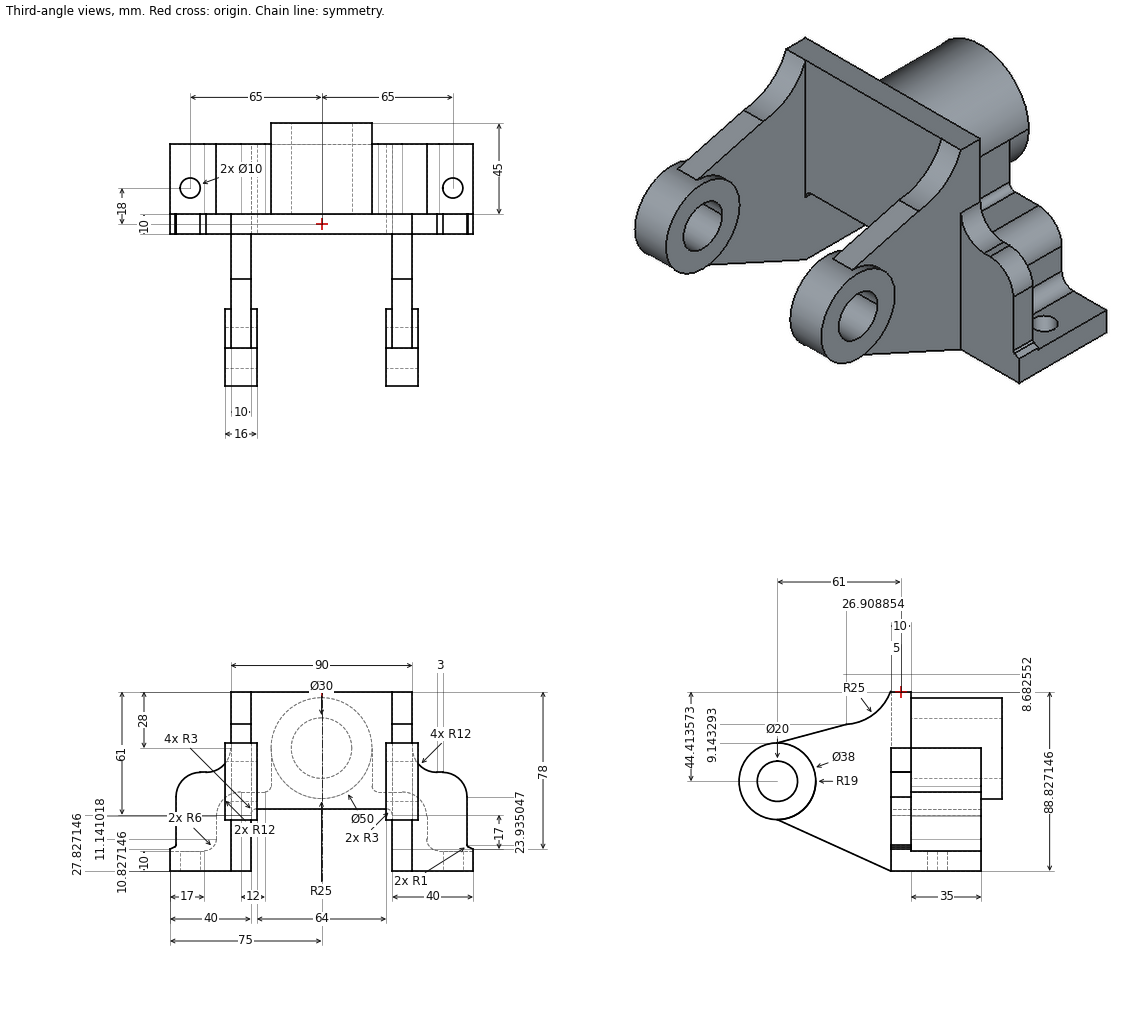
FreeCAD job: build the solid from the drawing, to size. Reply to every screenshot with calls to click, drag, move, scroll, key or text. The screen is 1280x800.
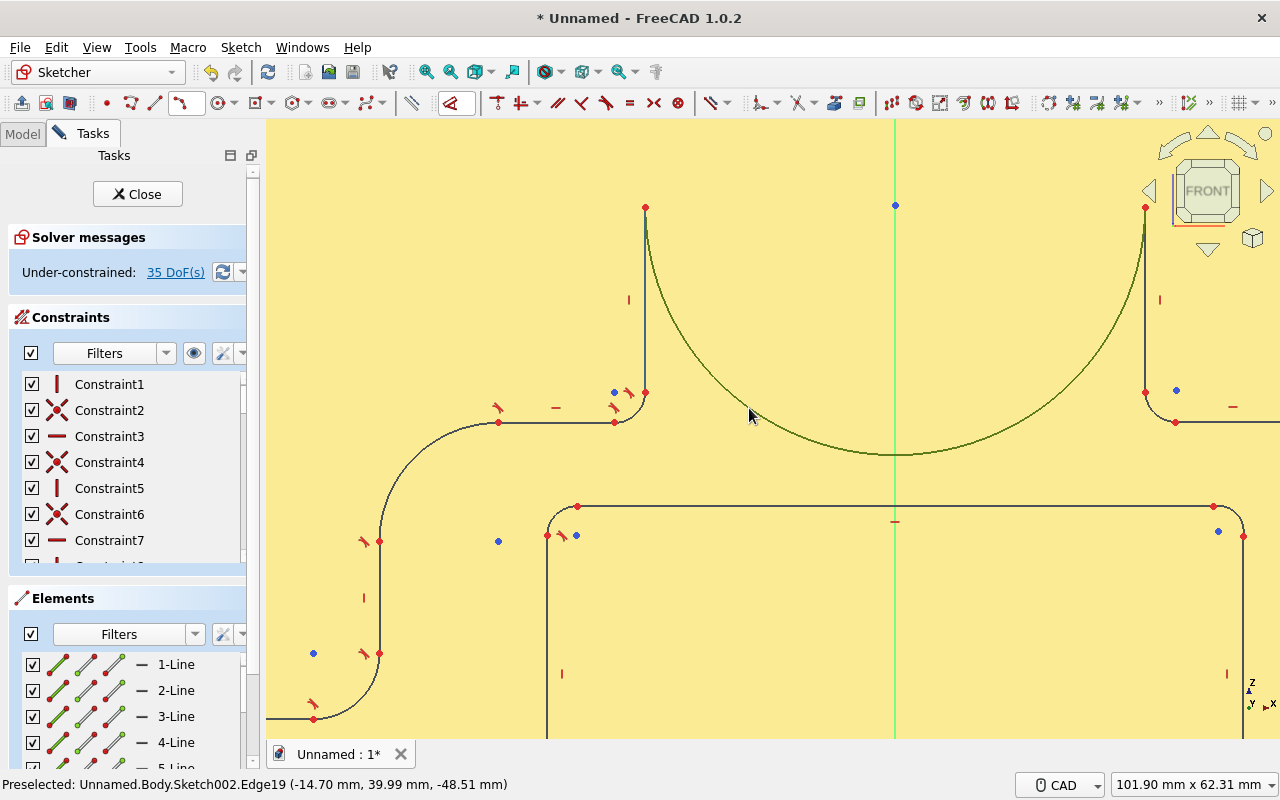
key(t)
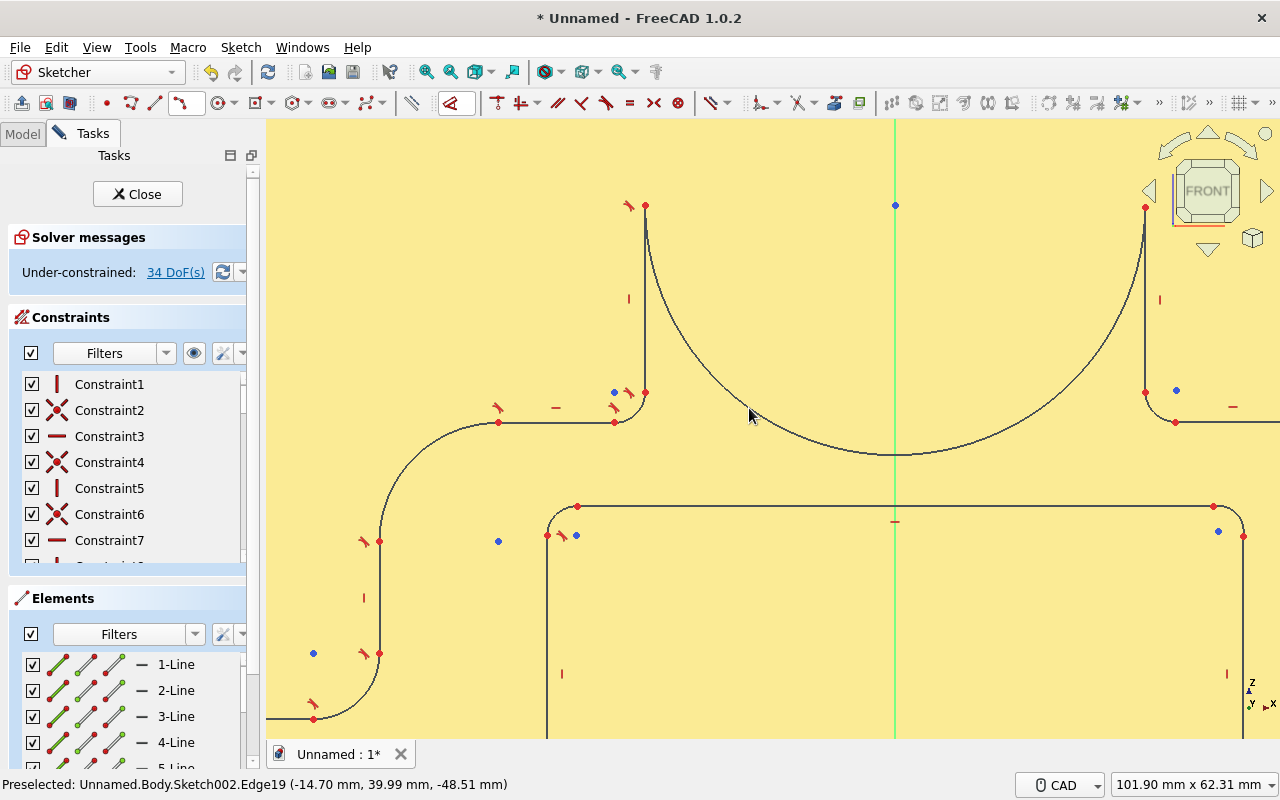
scroll(594, 465, down, 5)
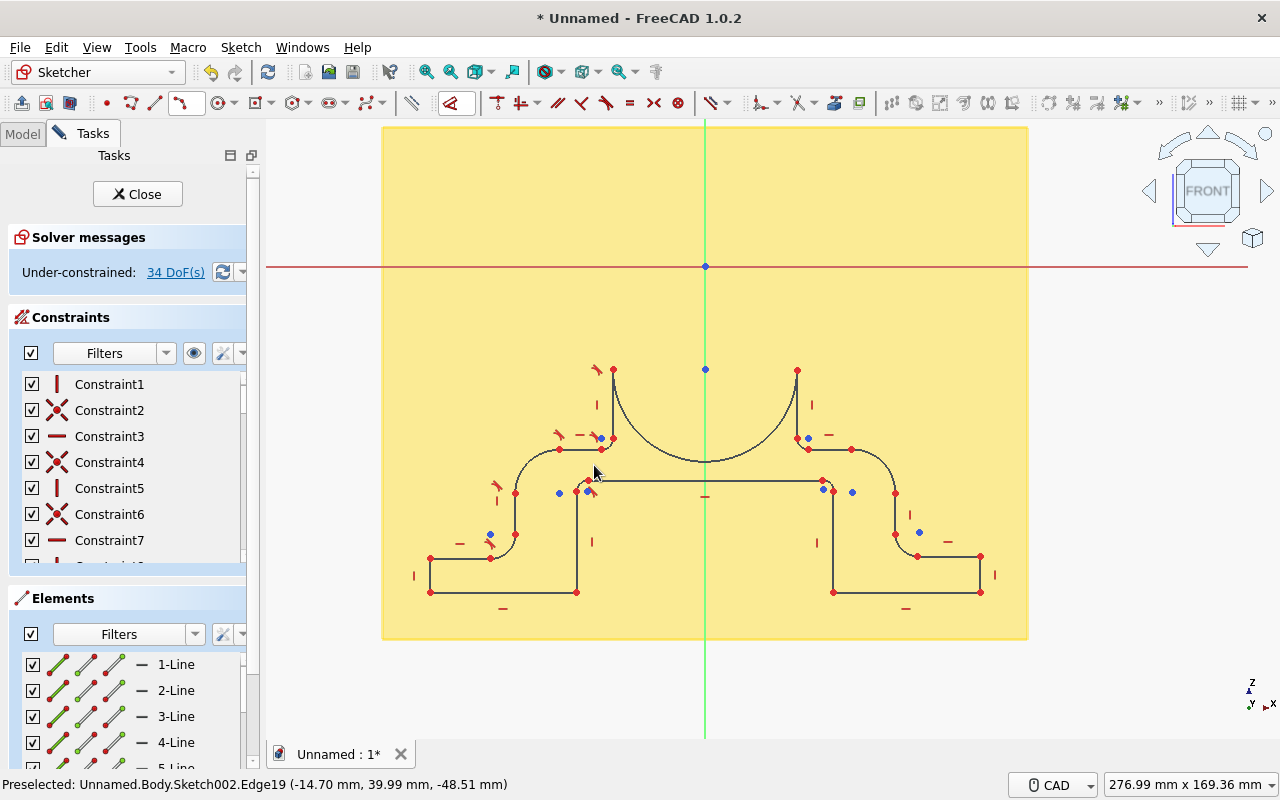
click(797, 418)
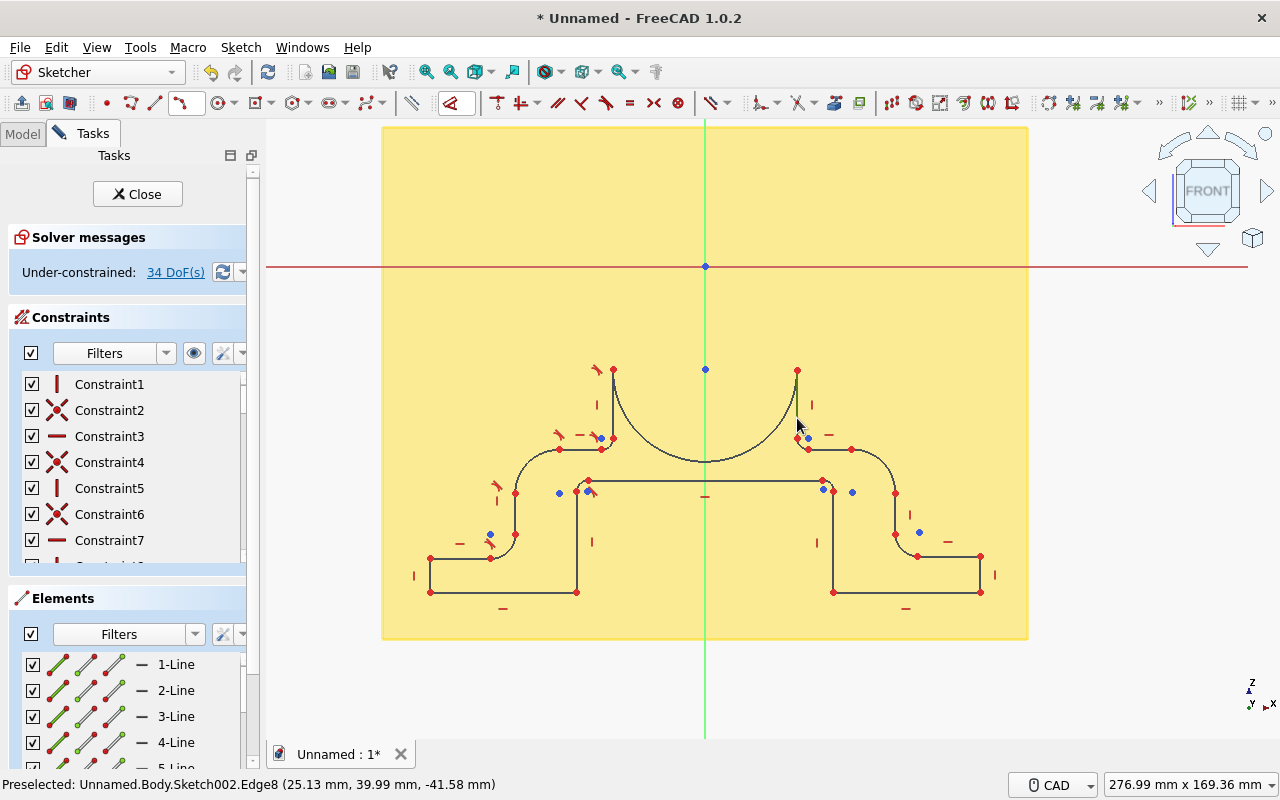
click(651, 444)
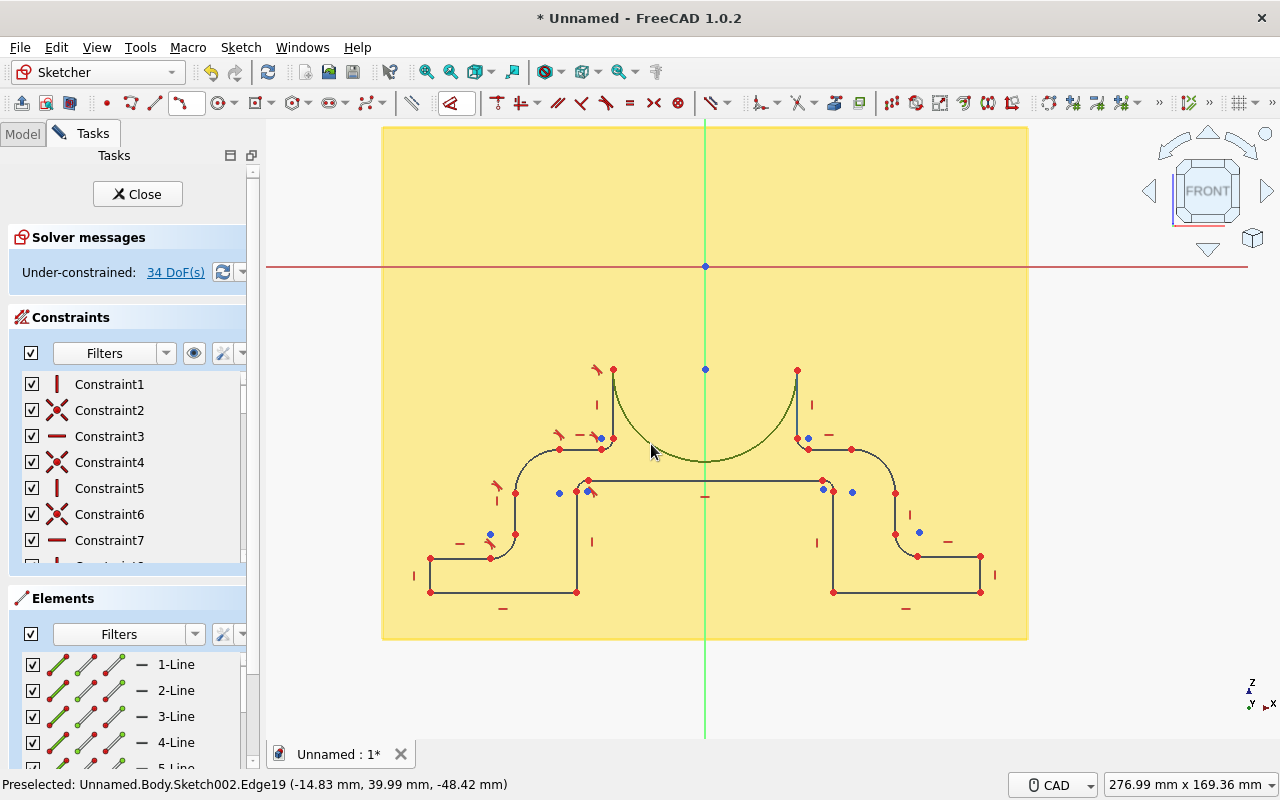
click(606, 104)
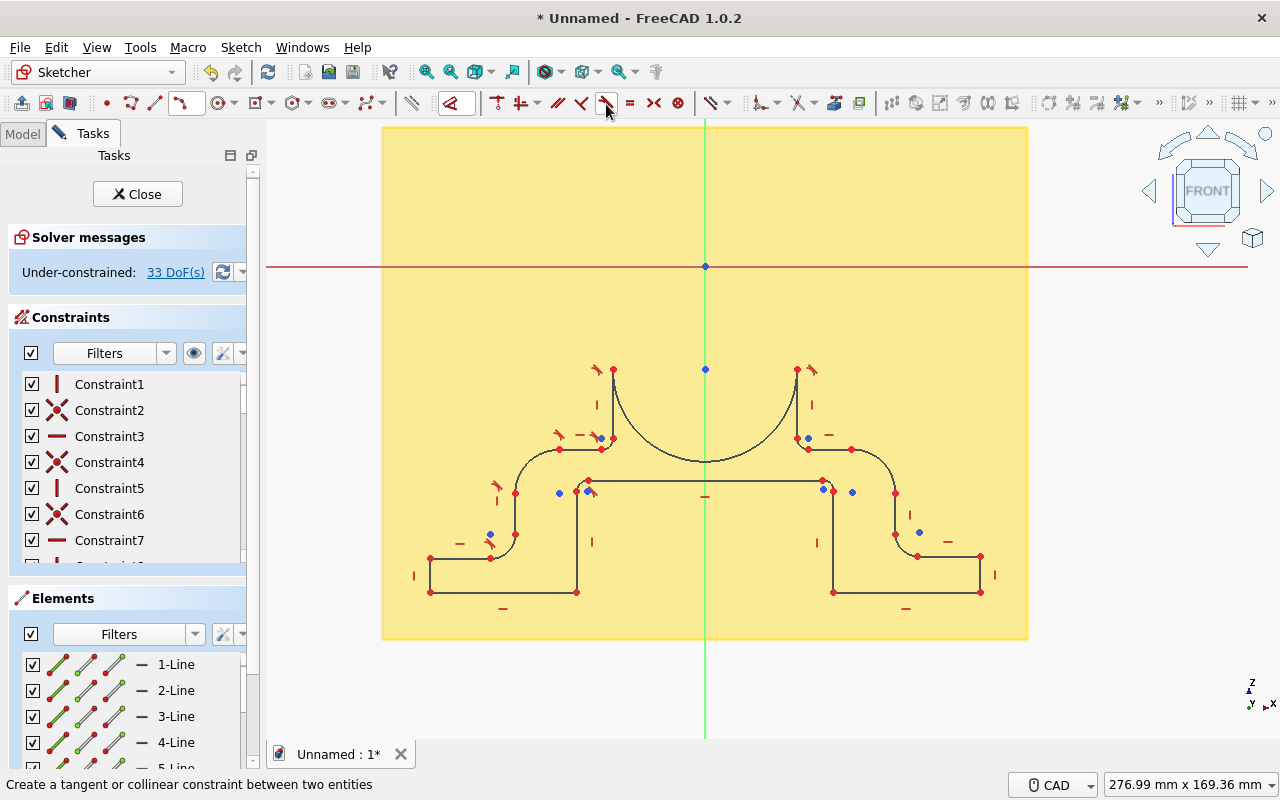
click(797, 418)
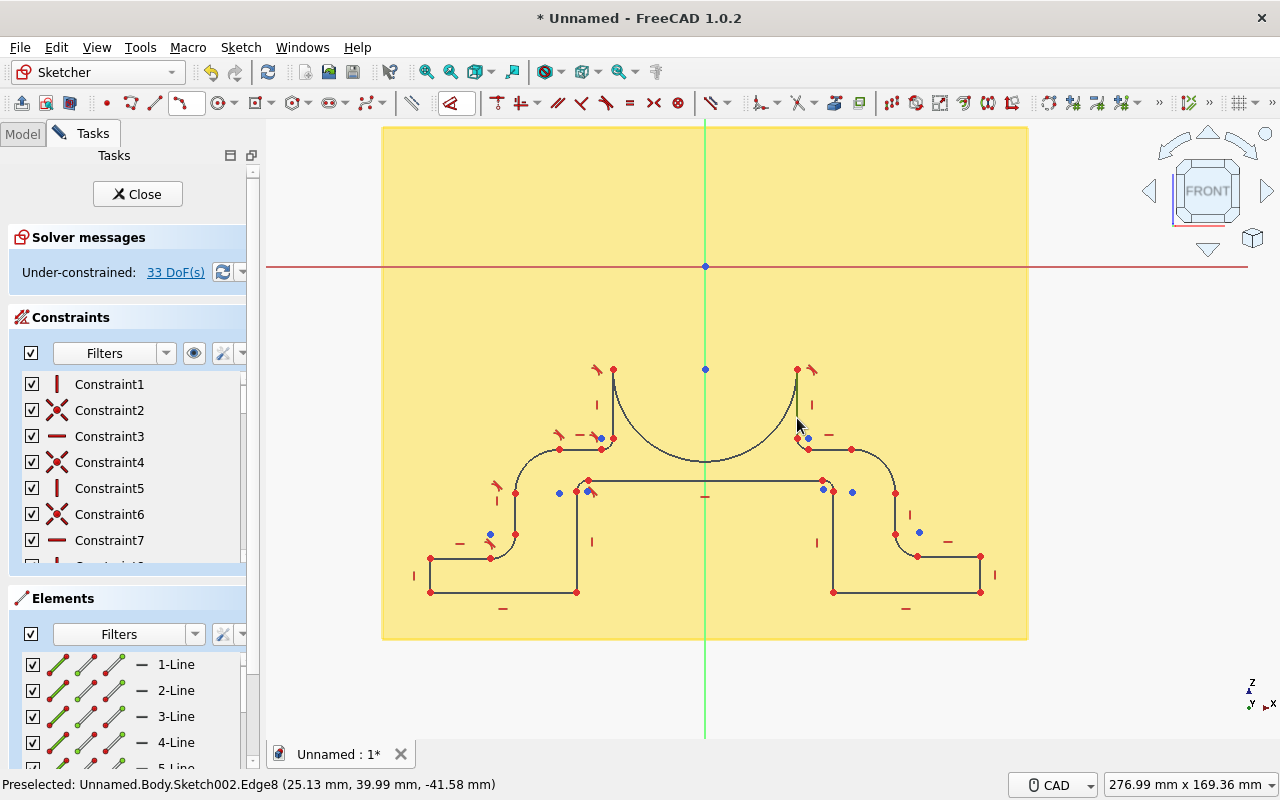
scroll(800, 446, up, 3)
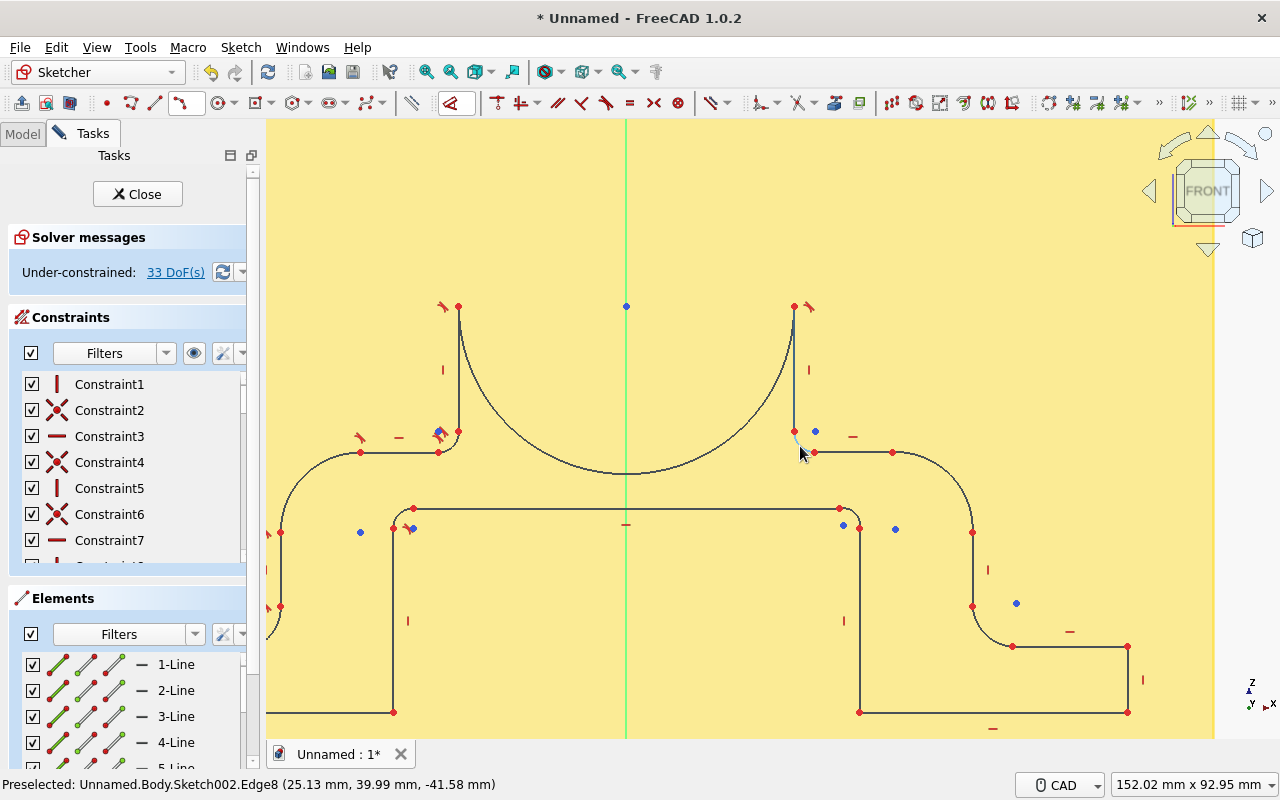
click(800, 446)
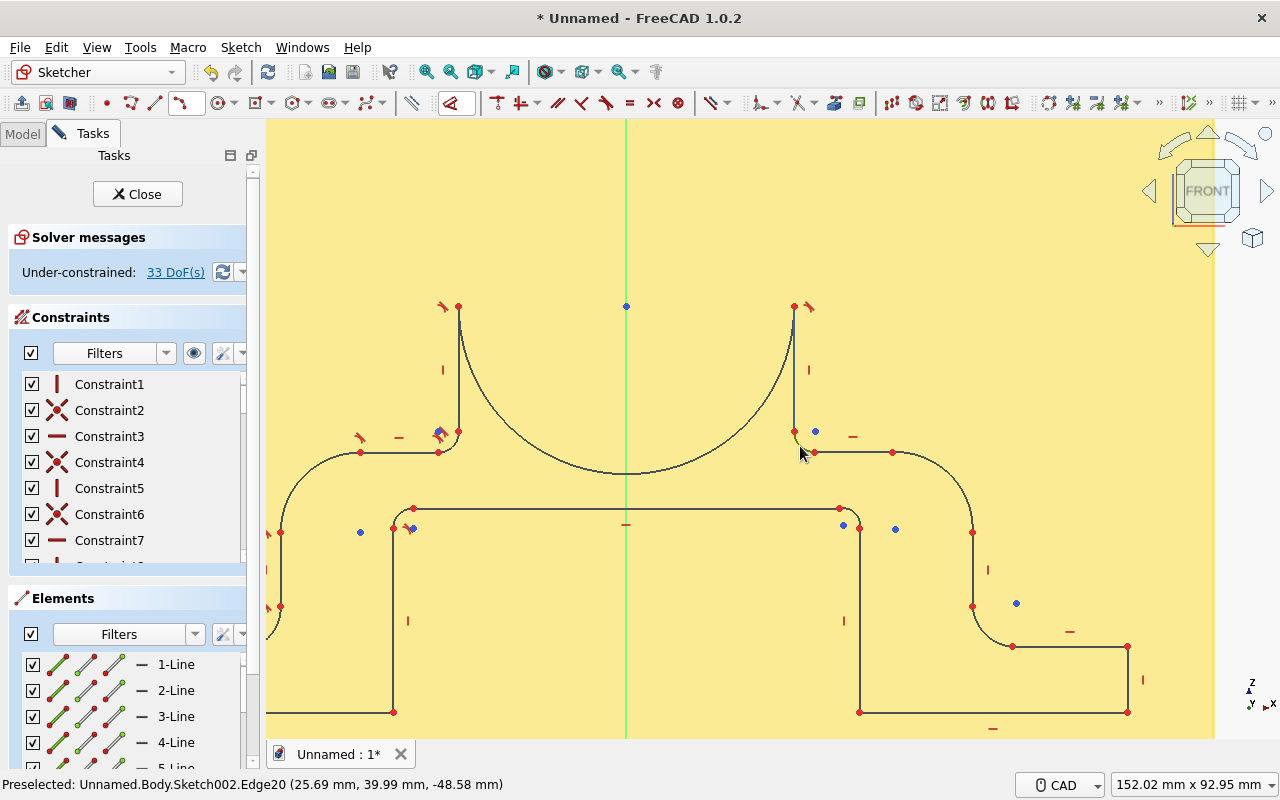
key(t)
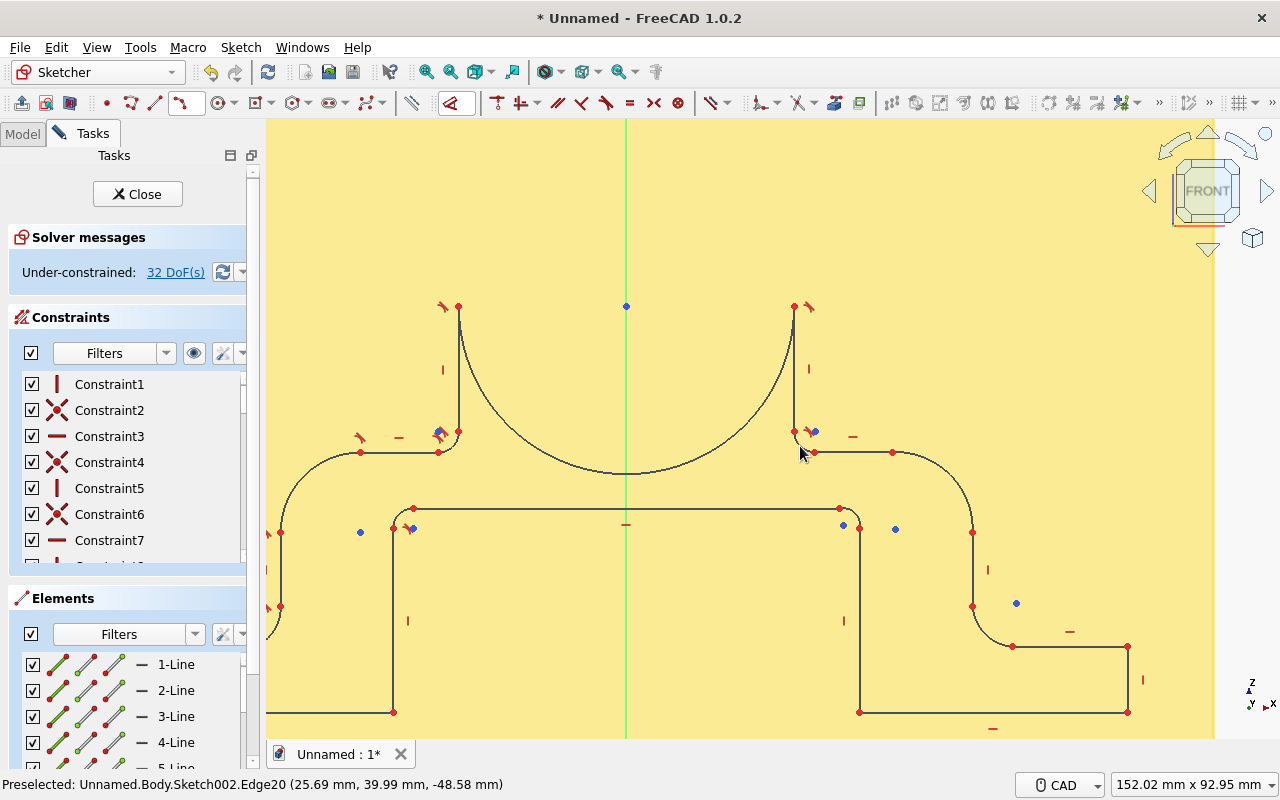
click(838, 452)